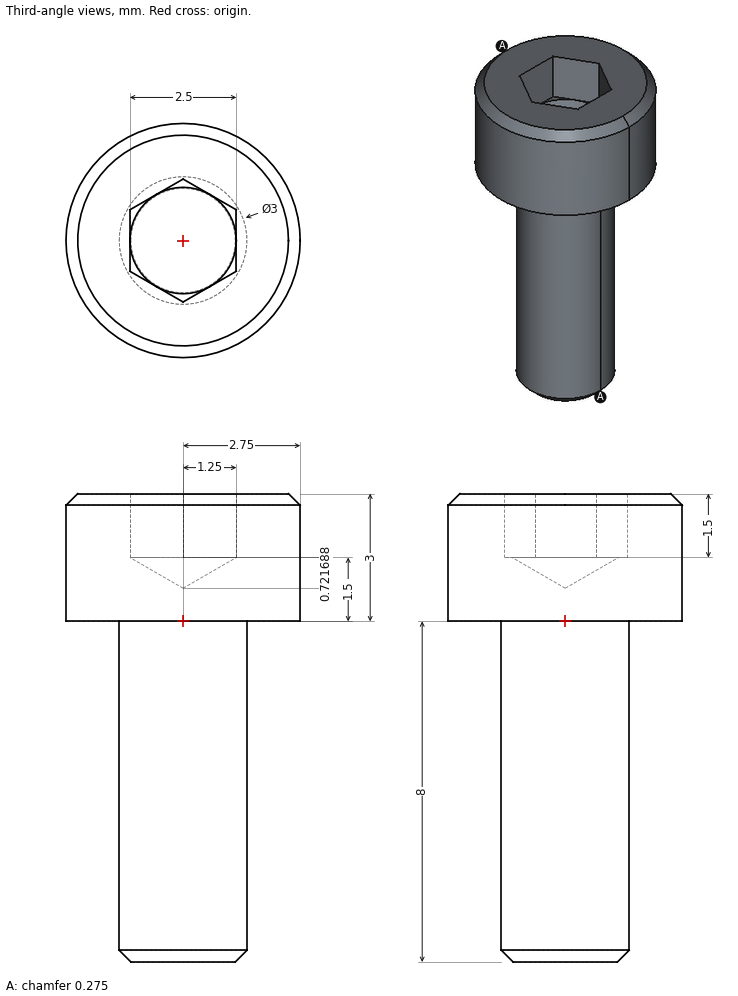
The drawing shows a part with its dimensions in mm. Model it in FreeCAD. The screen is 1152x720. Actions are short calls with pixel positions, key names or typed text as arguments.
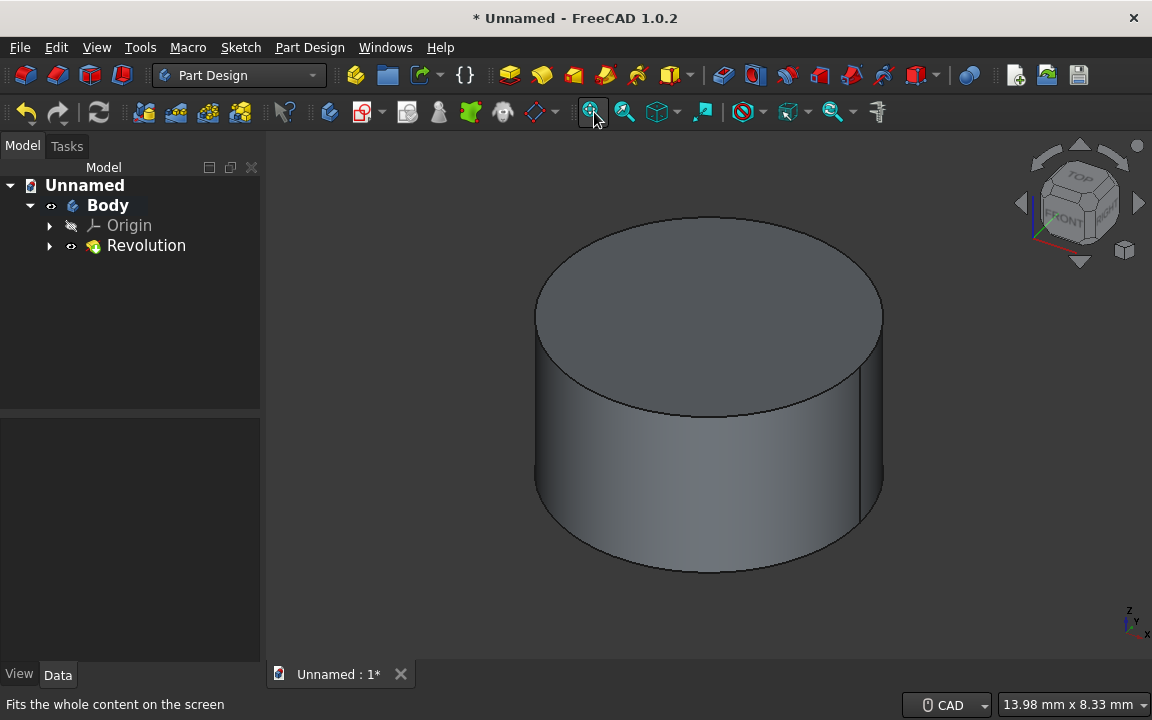
key(5)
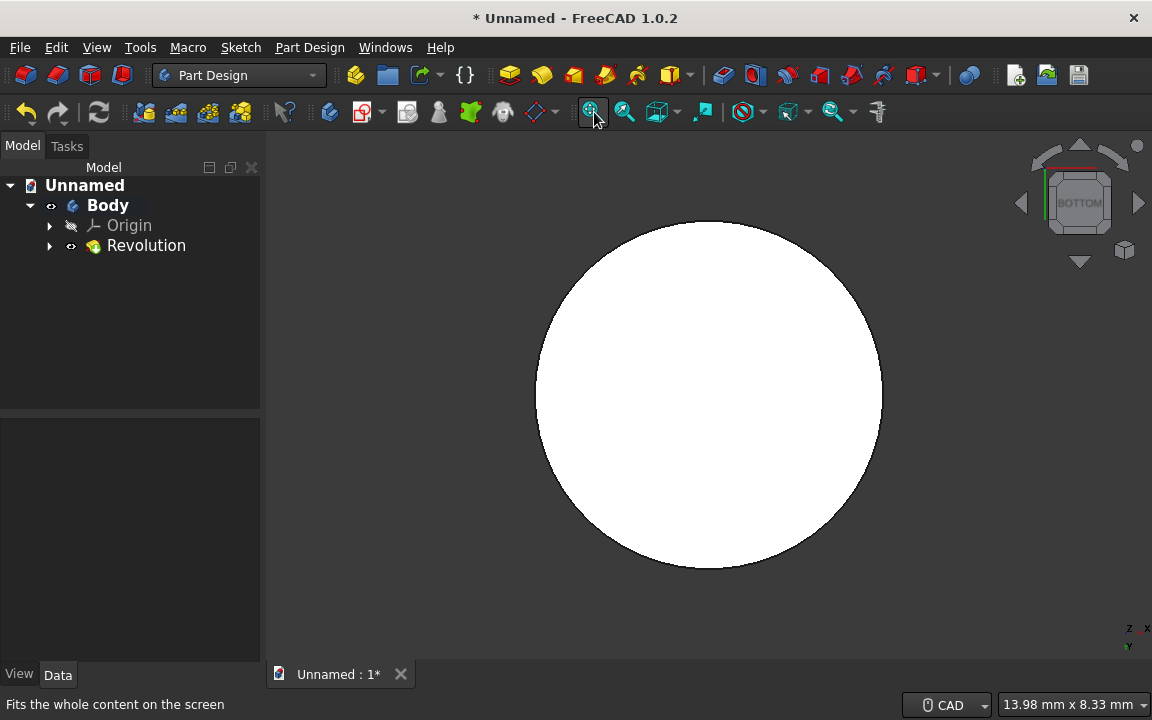
click(709, 394)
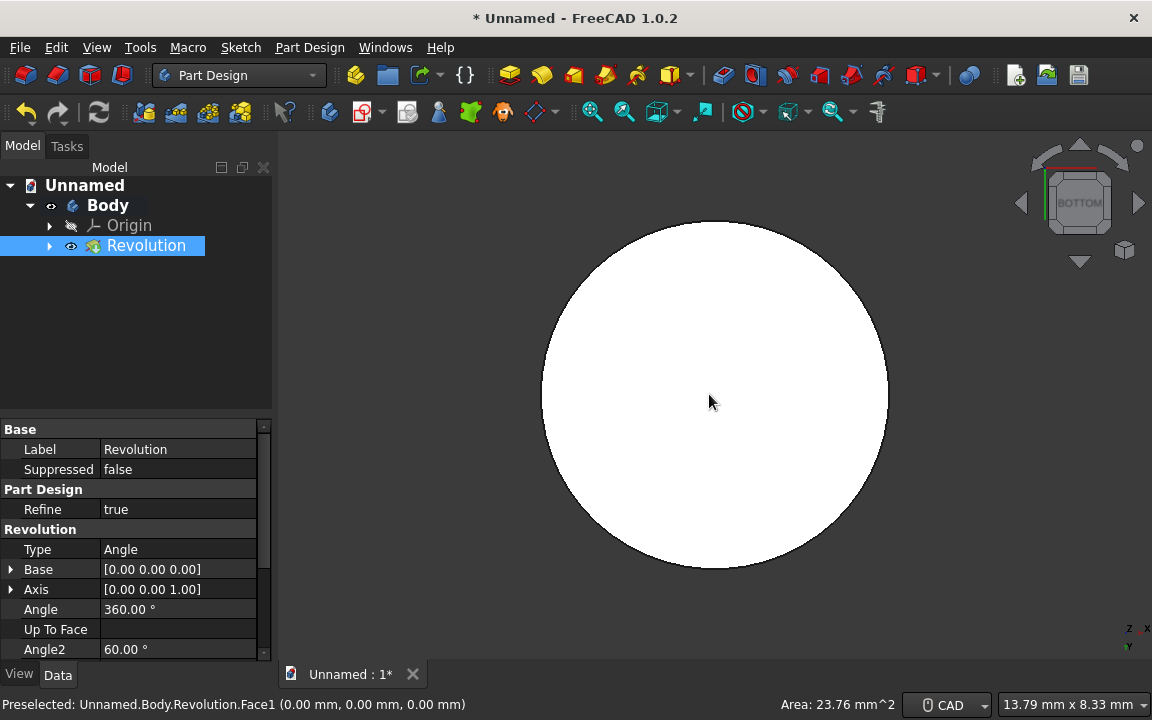
click(362, 112)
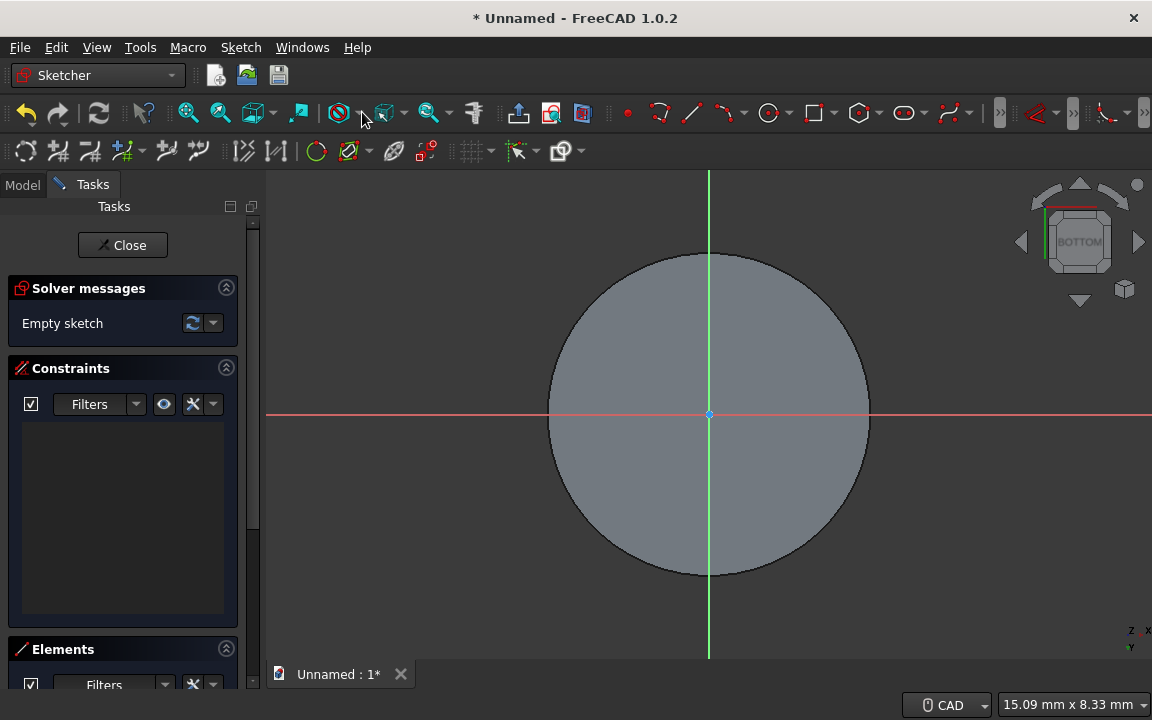
scroll(792, 415, up, 3)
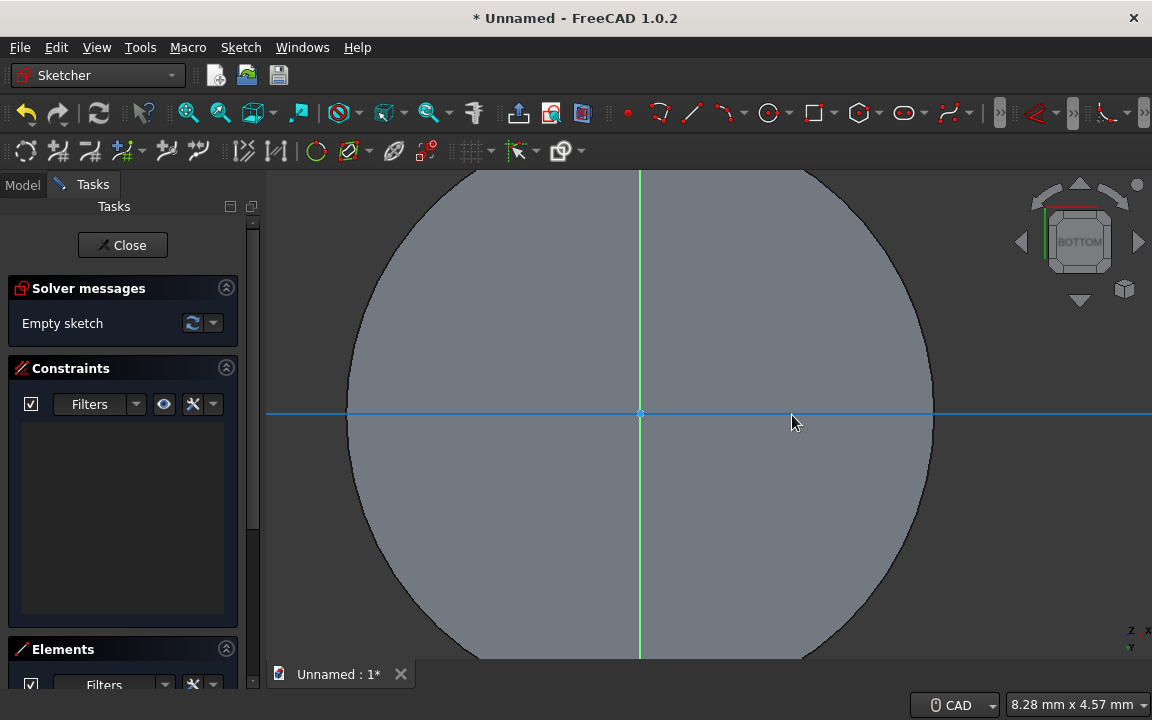
click(770, 114)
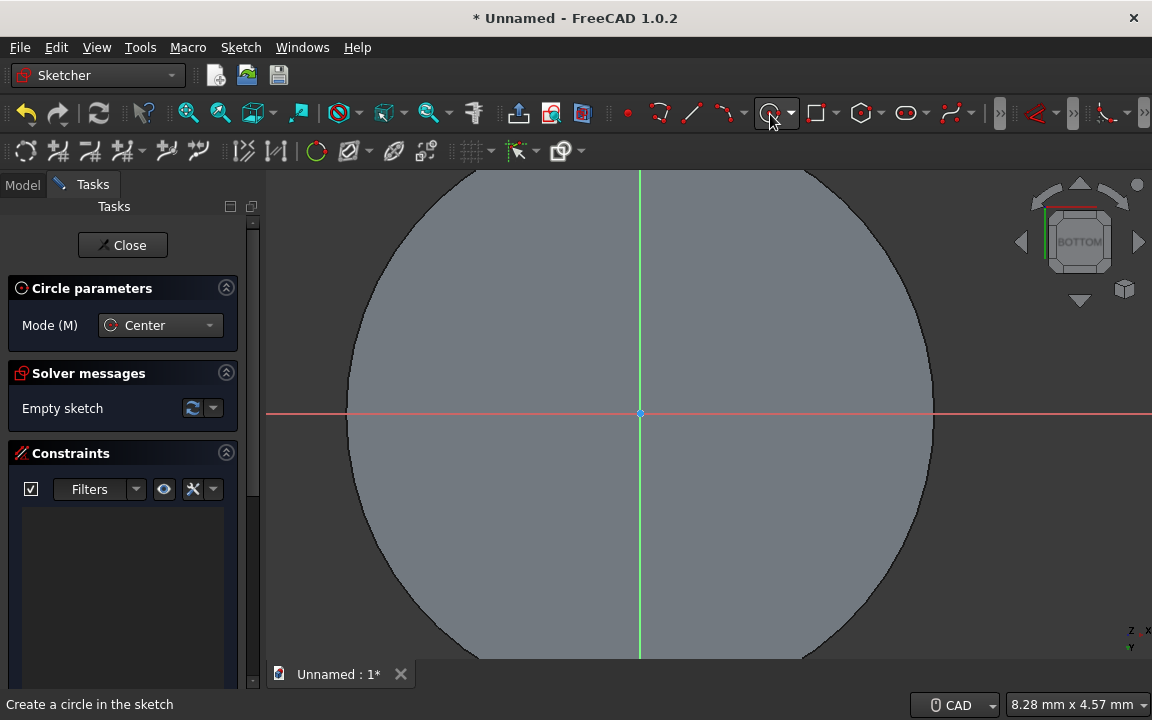
click(640, 414)
move(754, 300)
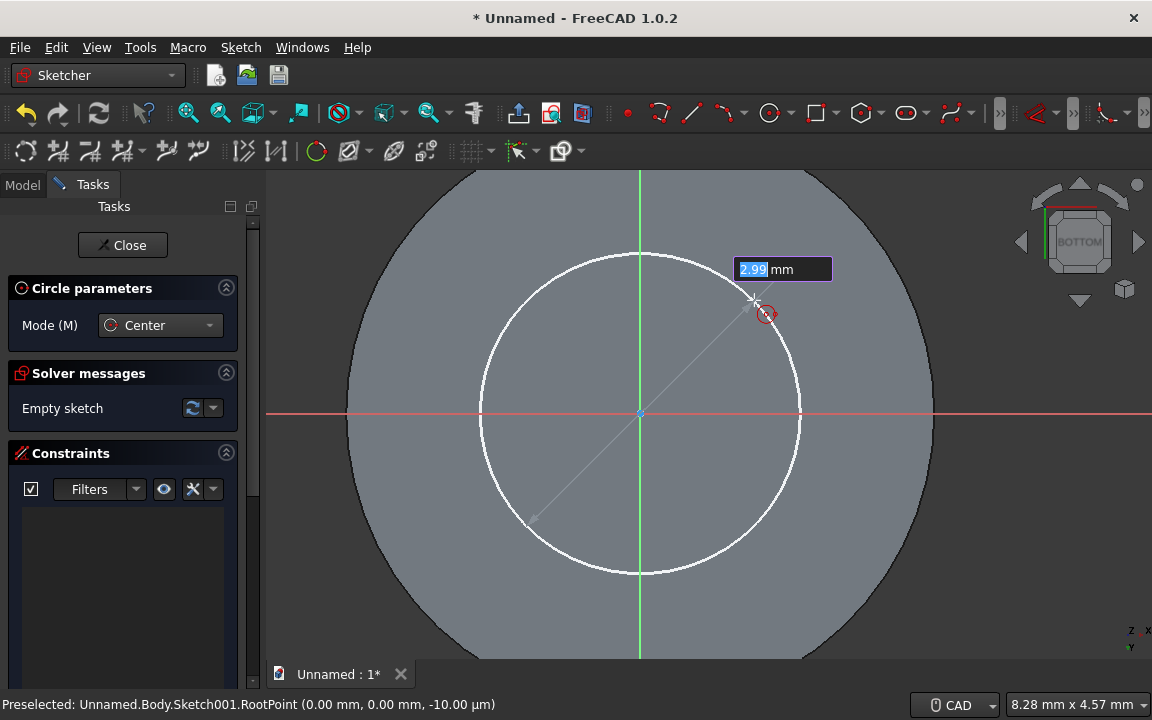
text(3)
key(Return)
key(Escape)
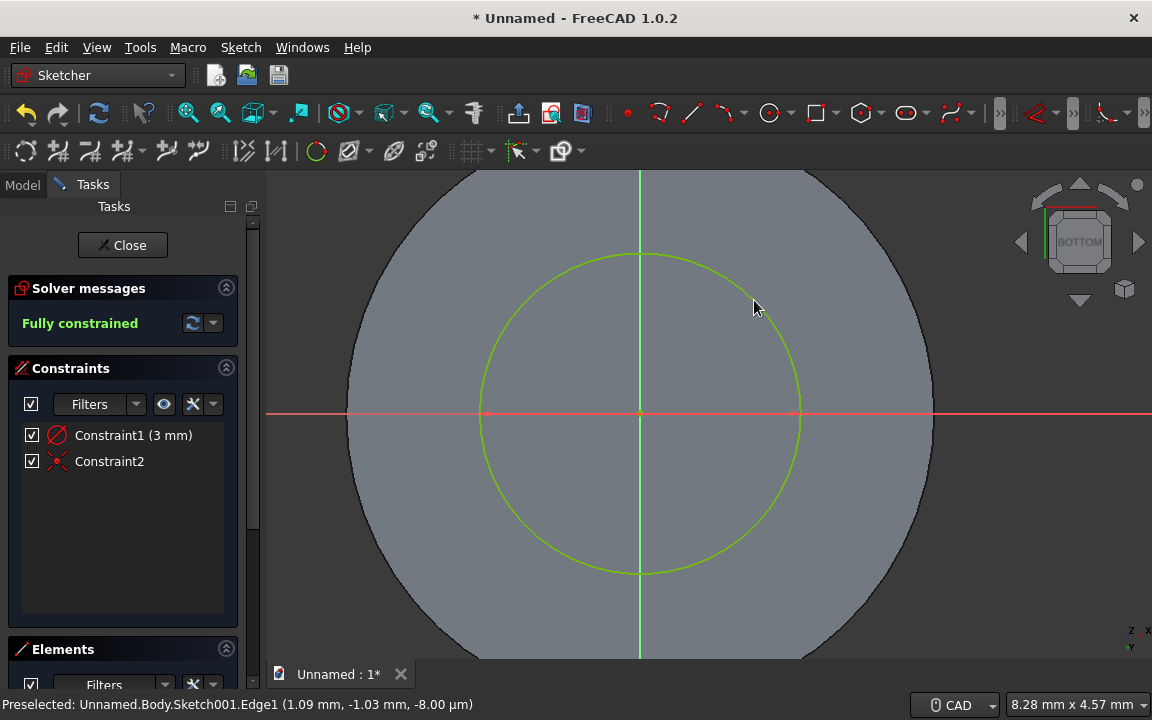
click(123, 245)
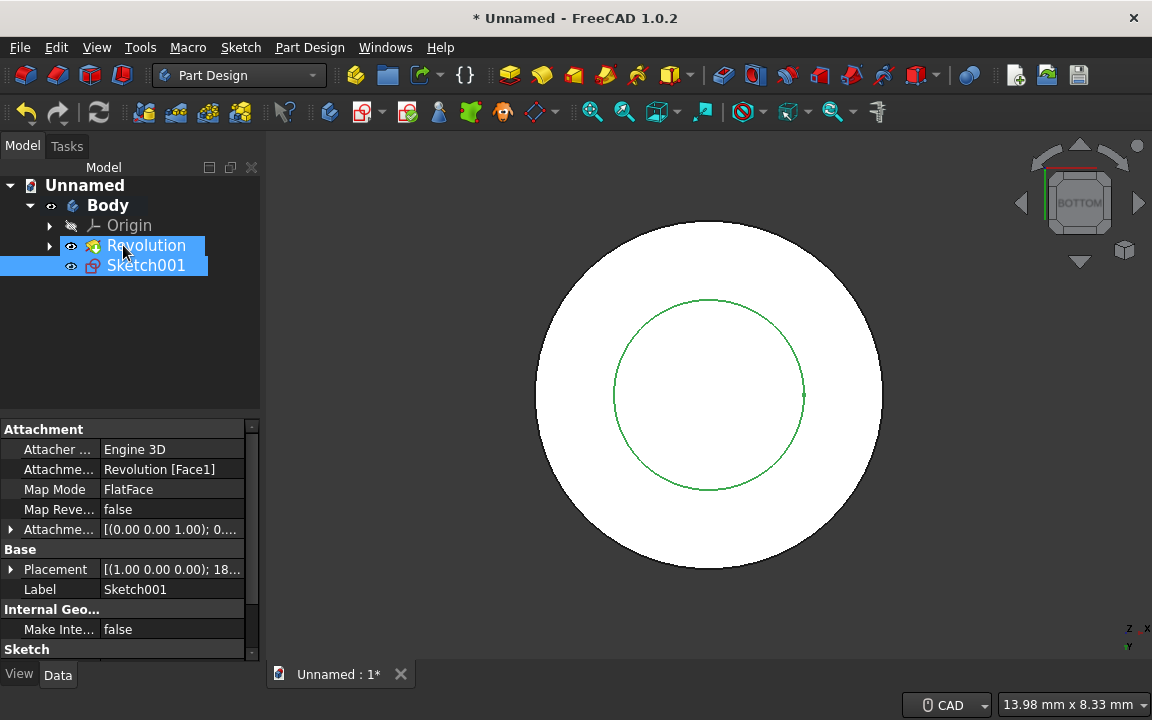
click(510, 76)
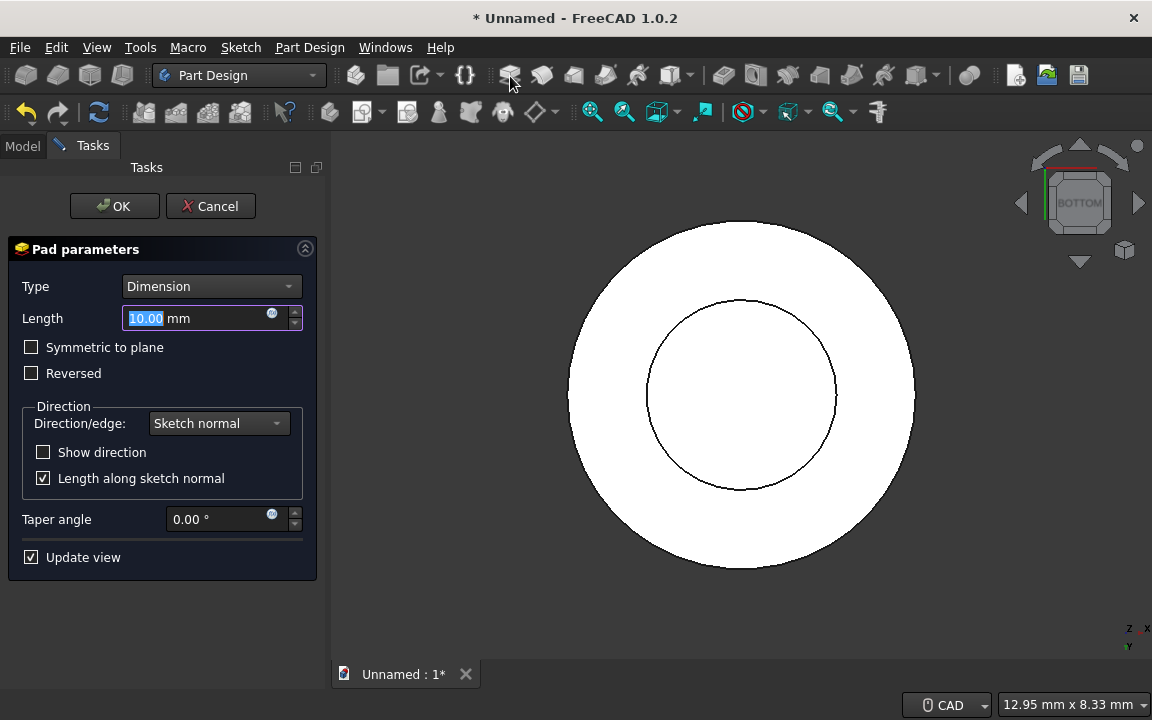
text(8)
key(Tab)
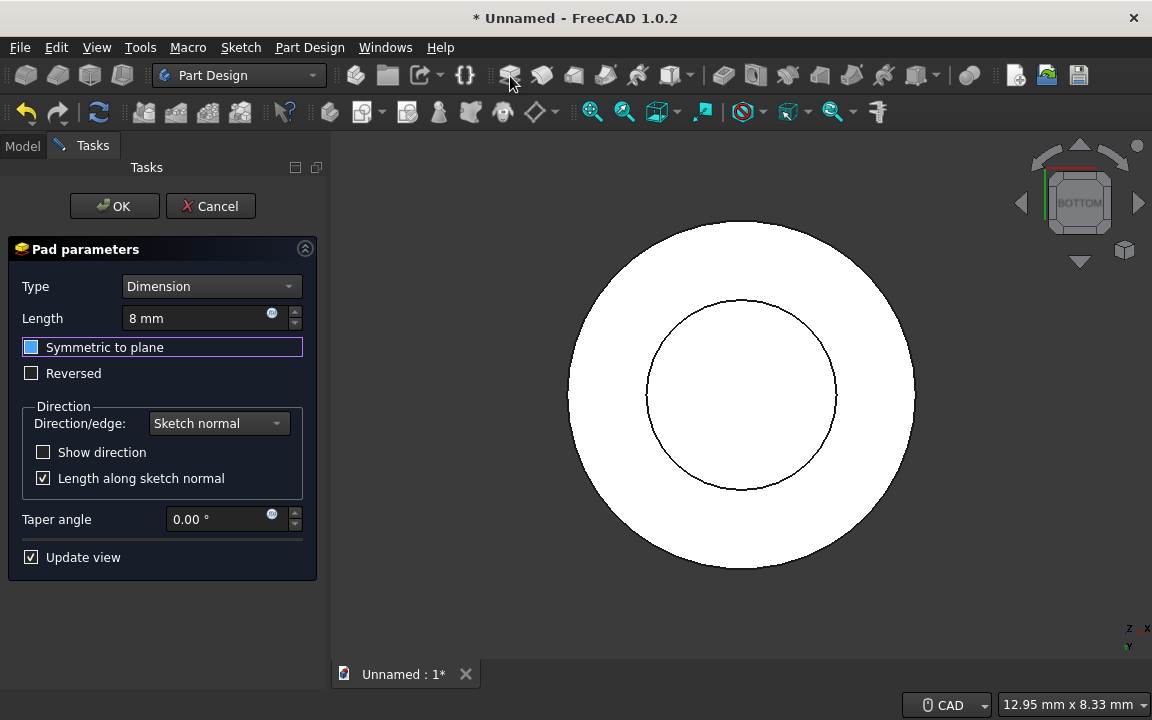
click(115, 206)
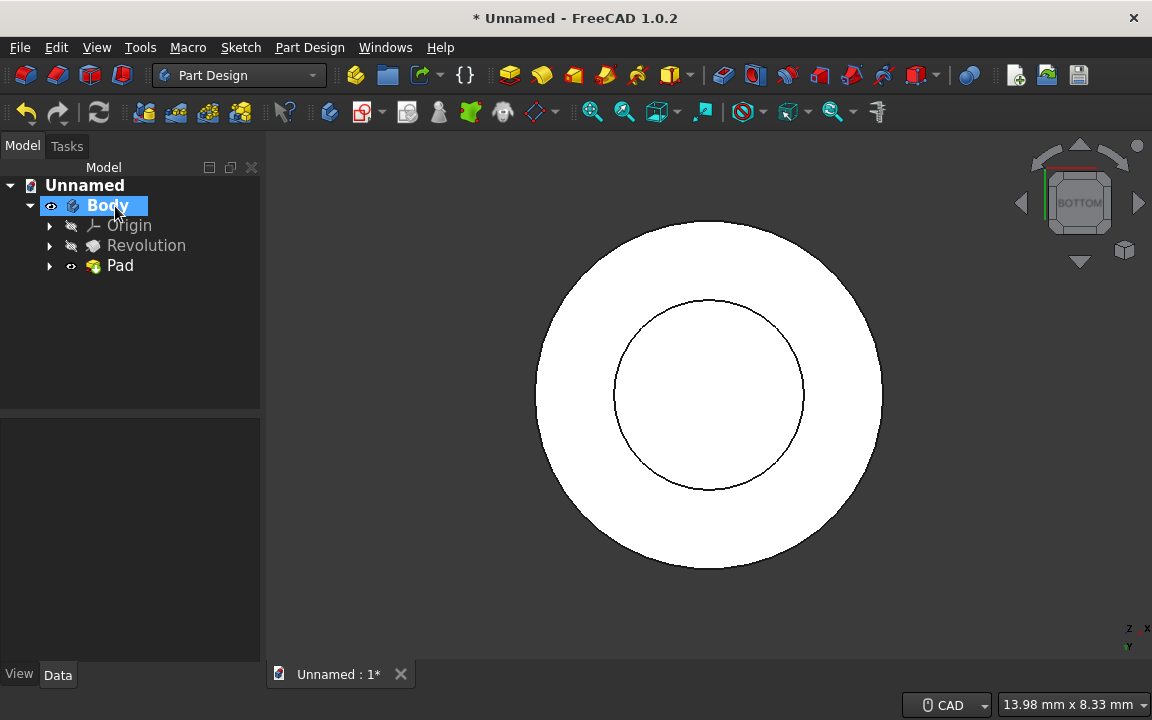
key(0)